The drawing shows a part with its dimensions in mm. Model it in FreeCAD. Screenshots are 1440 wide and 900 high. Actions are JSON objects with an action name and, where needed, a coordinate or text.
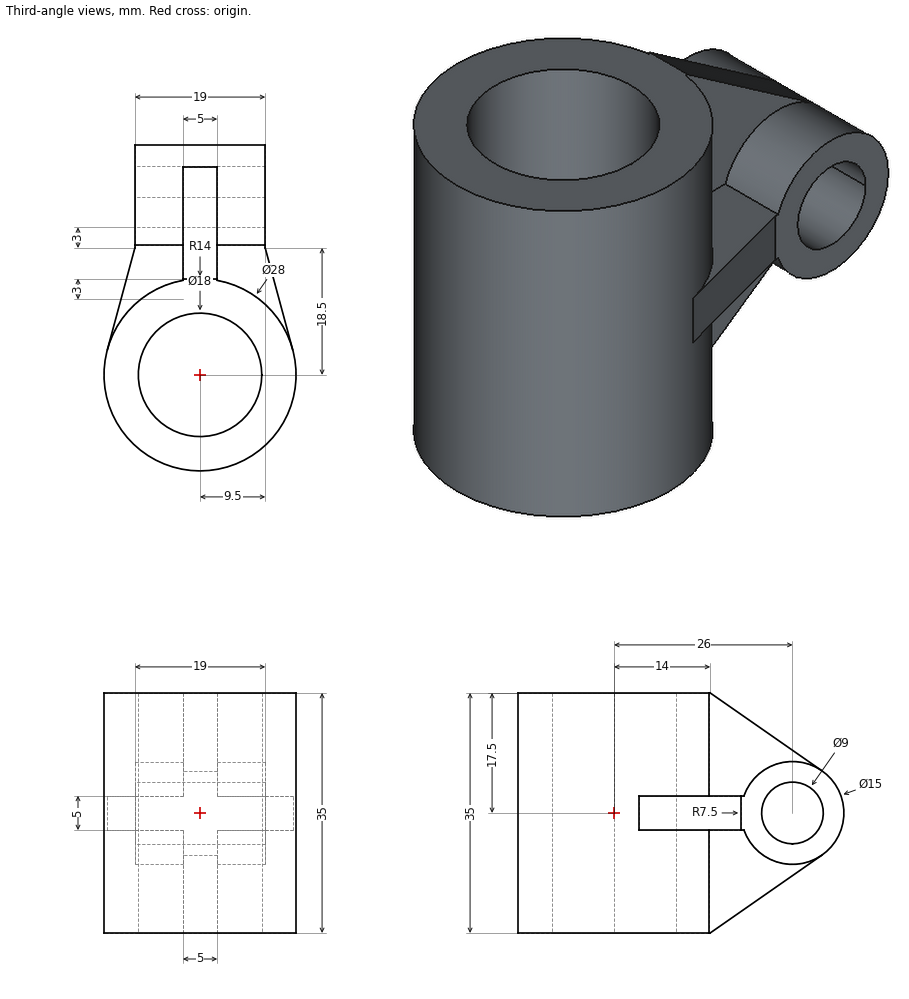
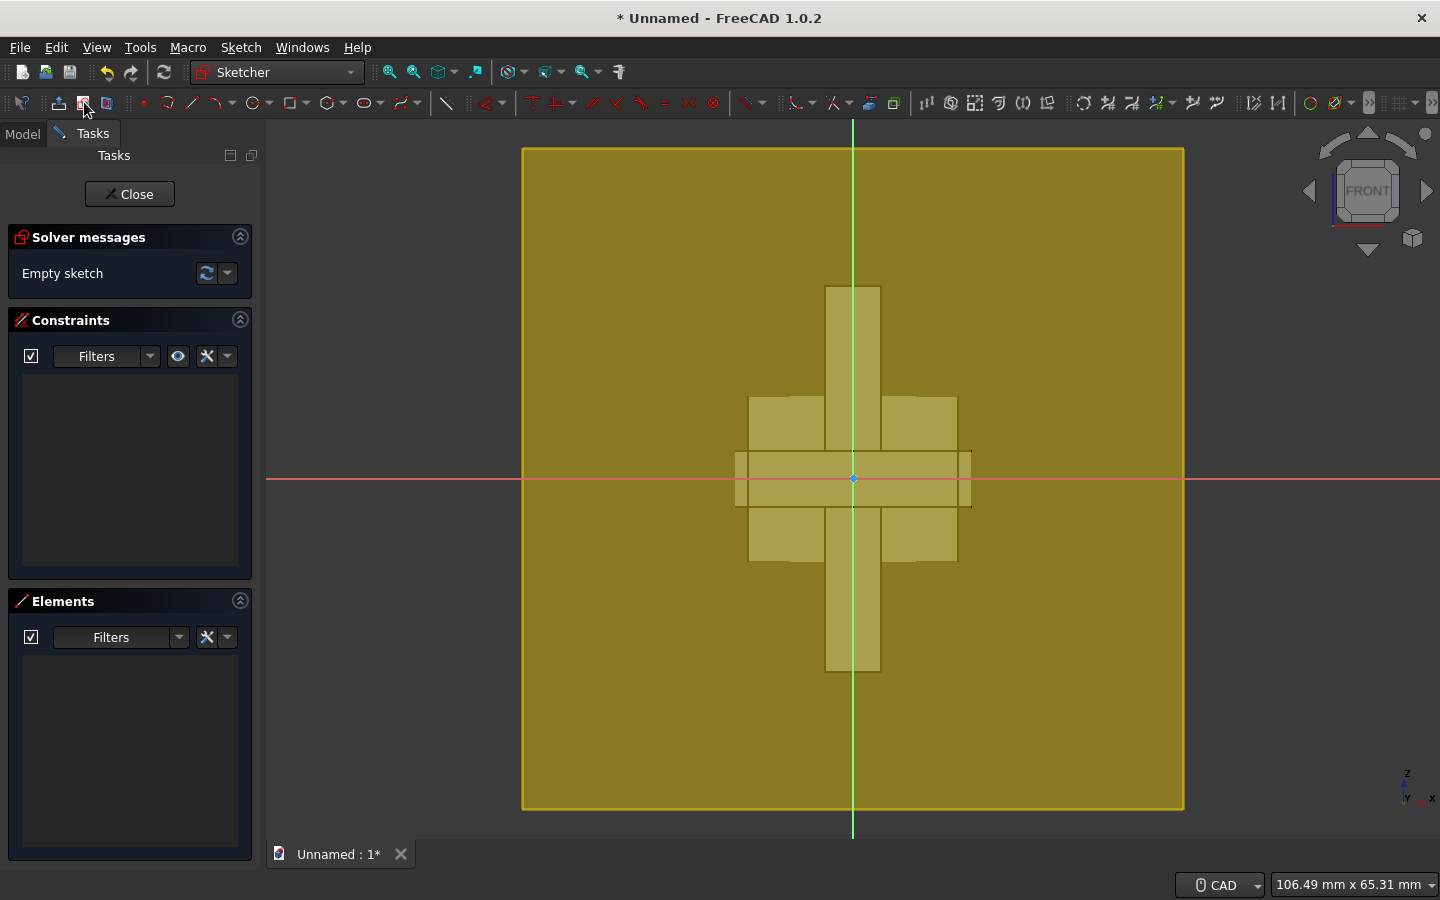
{"action": "key", "text": "g v"}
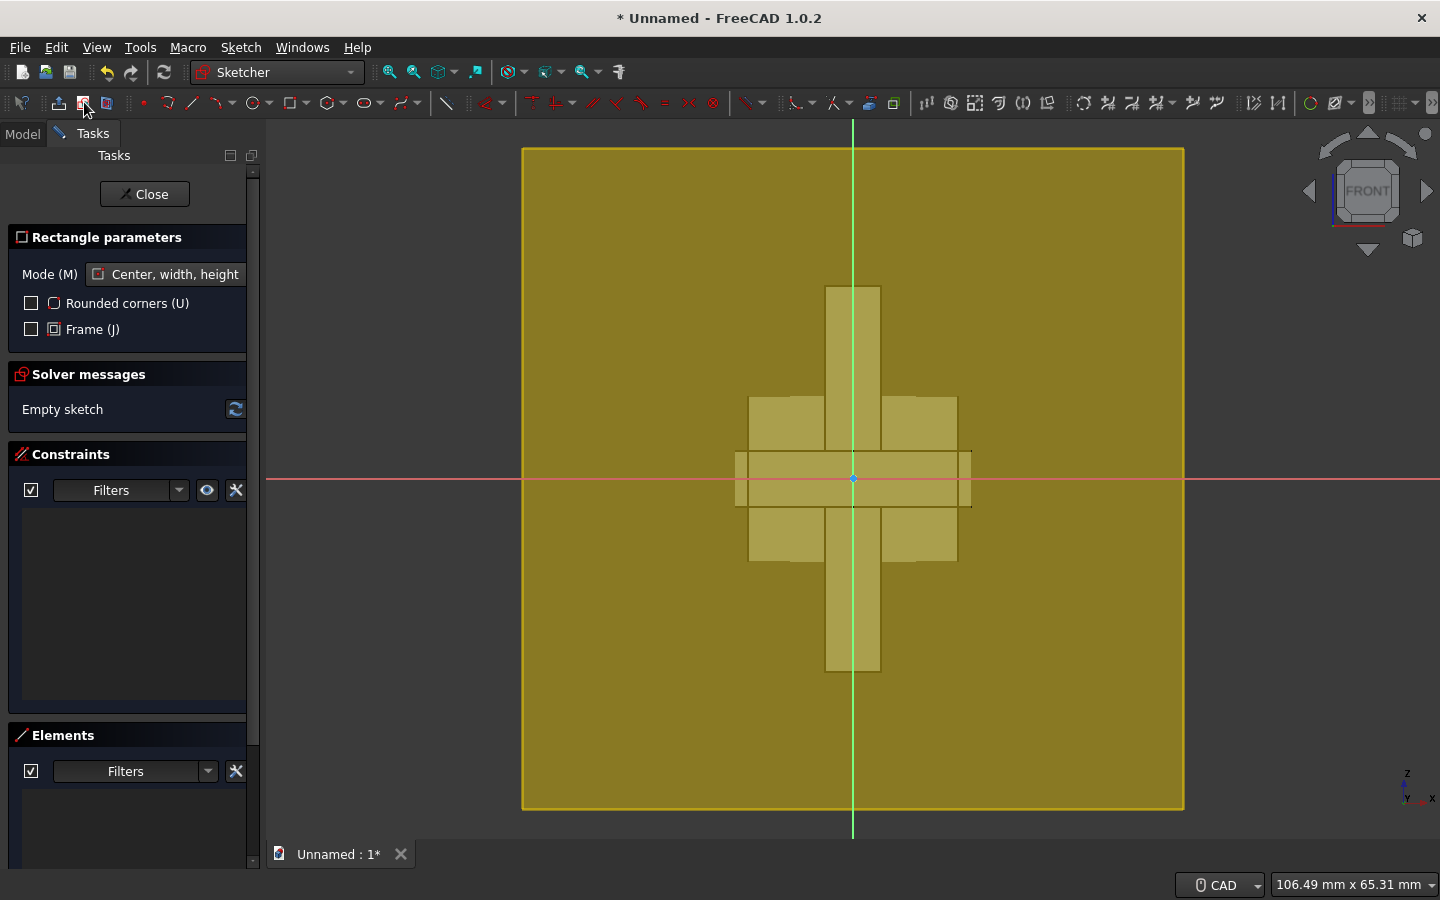
{"action": "left_click", "coordinate": [853, 479]}
{"action": "left_click", "coordinate": [881, 286]}
{"action": "key", "text": "Escape"}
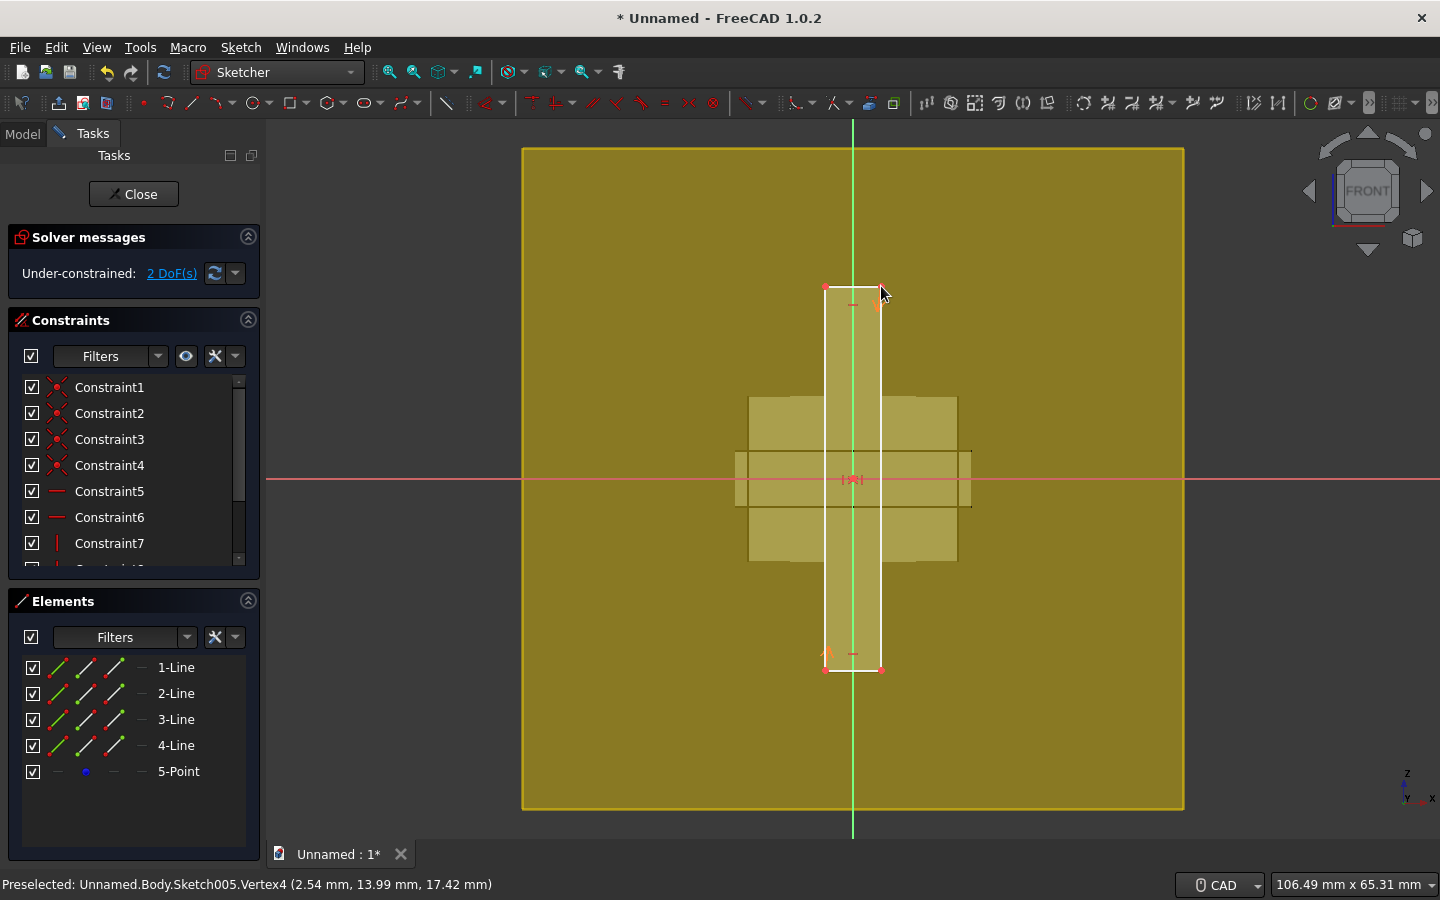
{"action": "left_click", "coordinate": [486, 104]}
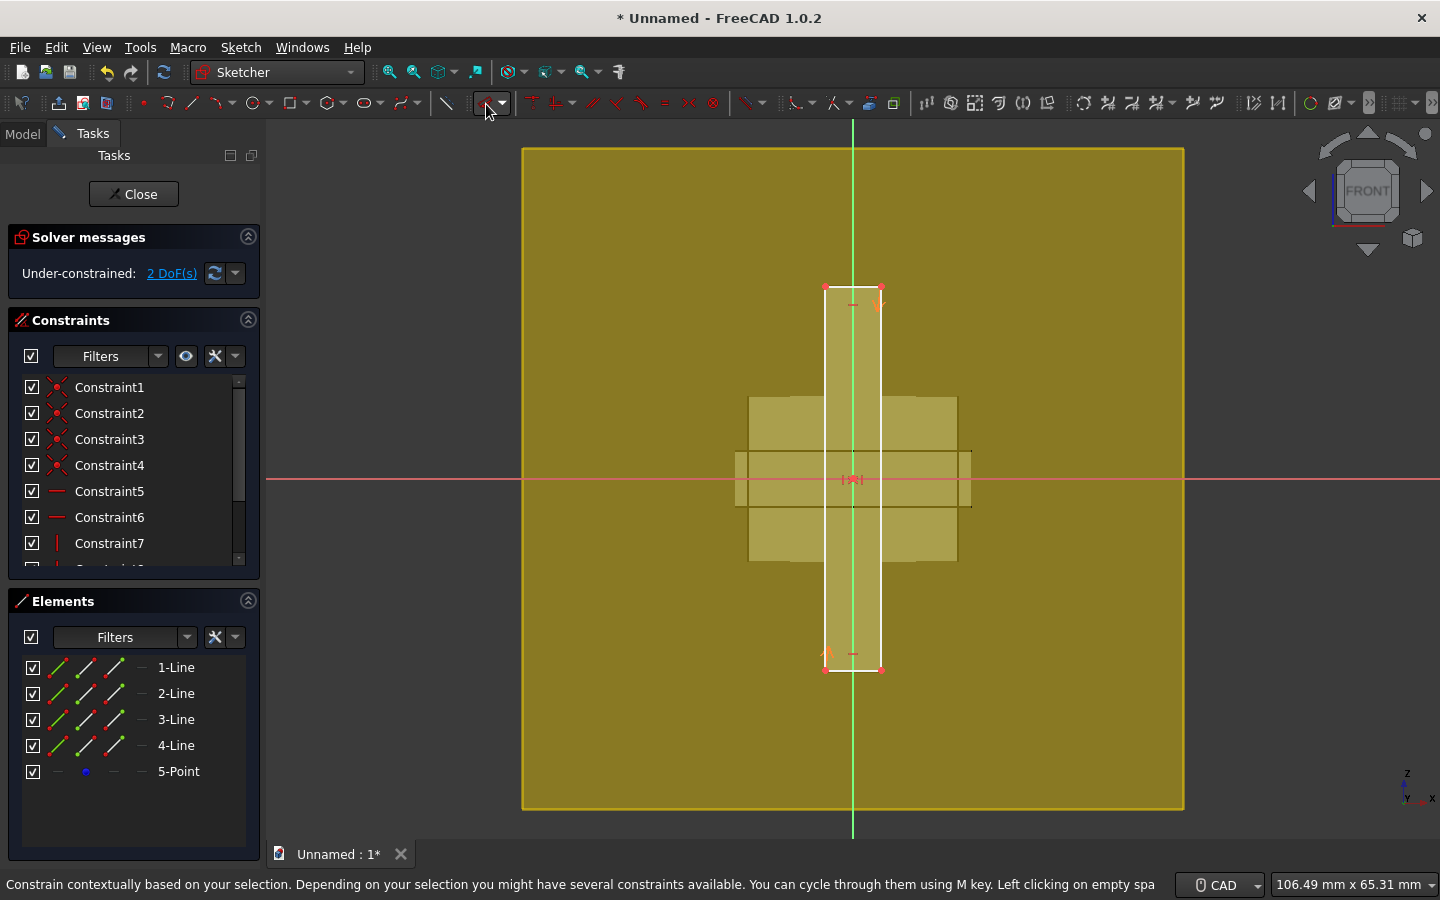
{"action": "scroll", "coordinate": [842, 671], "scroll_direction": "up", "scroll_amount": 2}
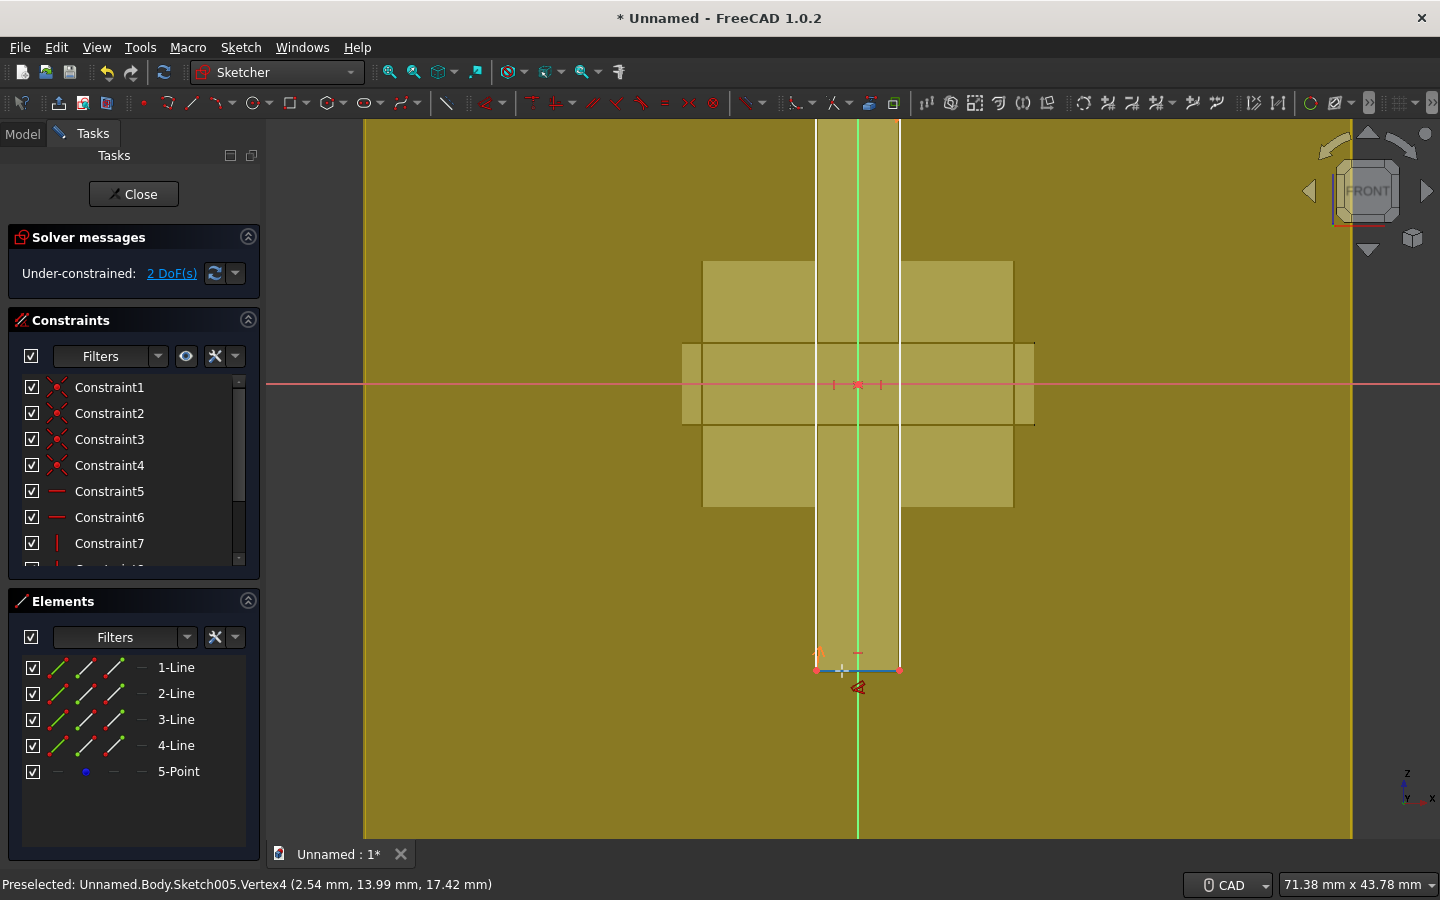
{"action": "left_click", "coordinate": [841, 671]}
{"action": "left_click", "coordinate": [839, 705]}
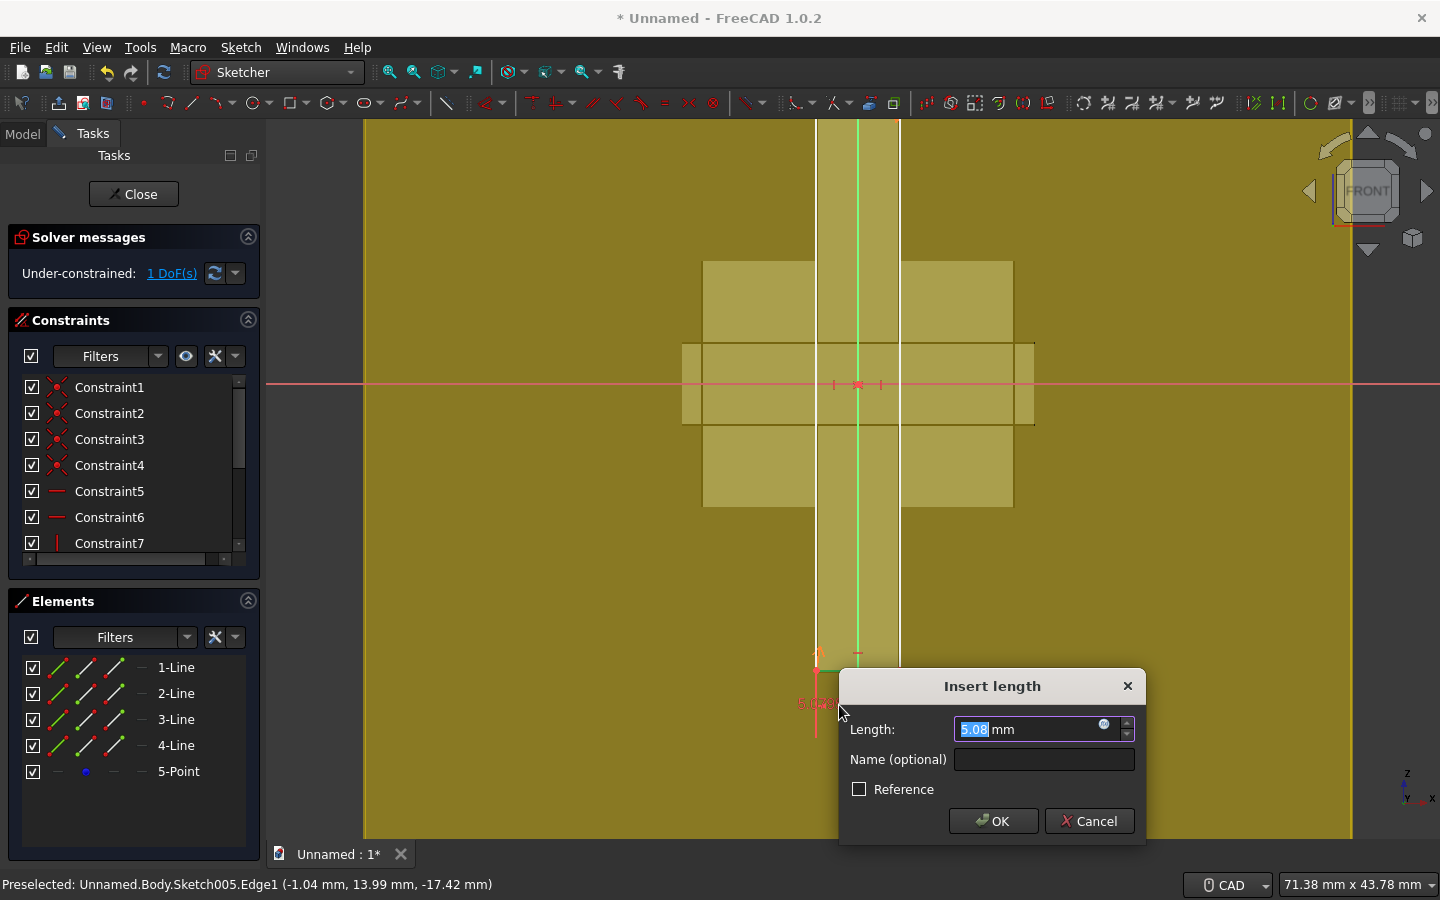
{"action": "type", "text": "5"}
{"action": "key", "text": "Return"}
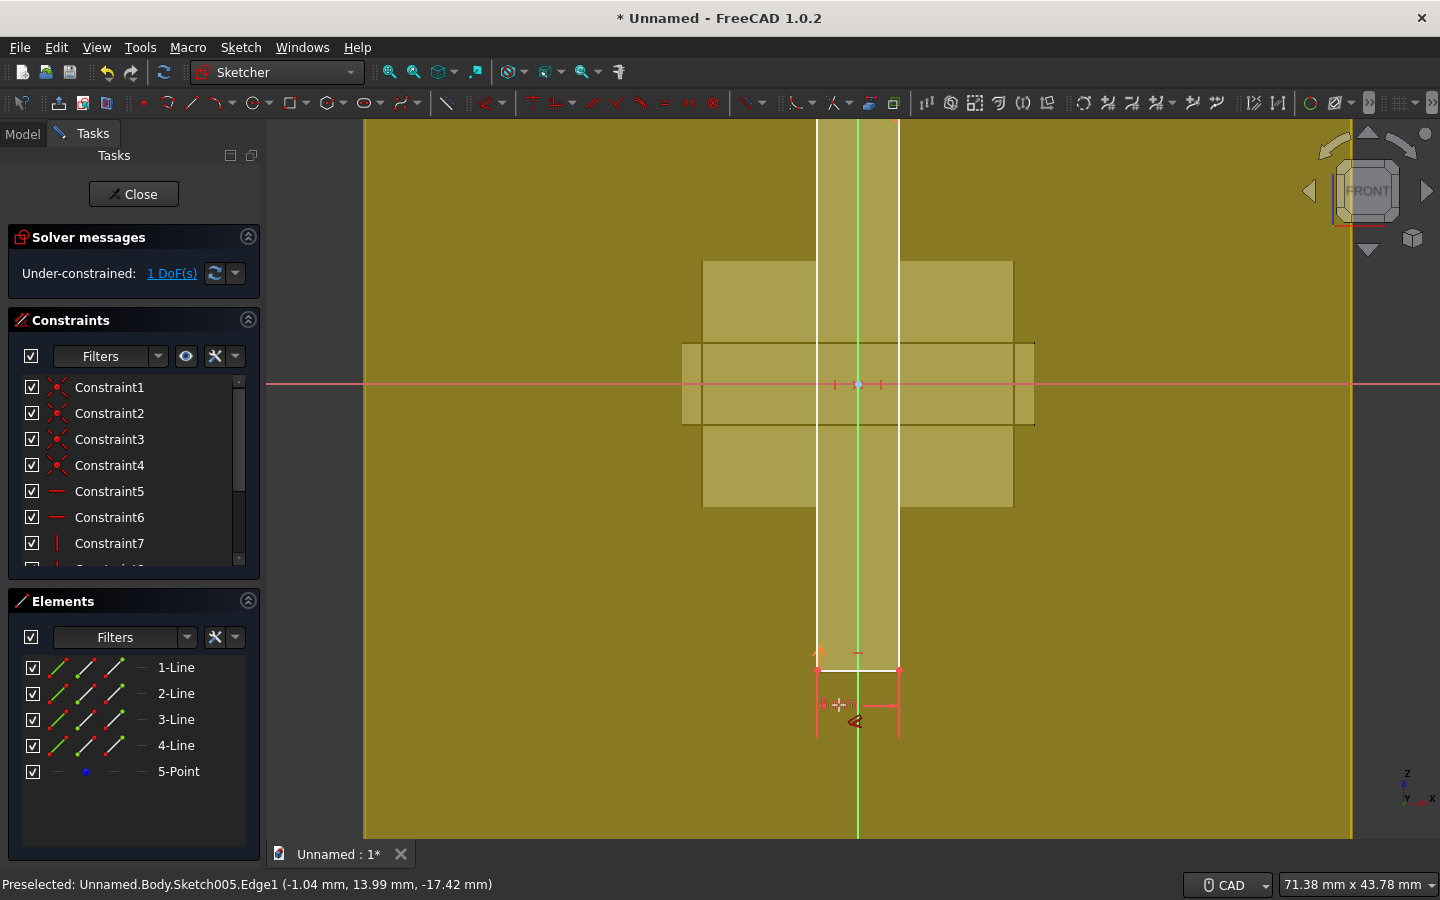
{"action": "left_click", "coordinate": [899, 499]}
{"action": "left_click", "coordinate": [933, 409]}